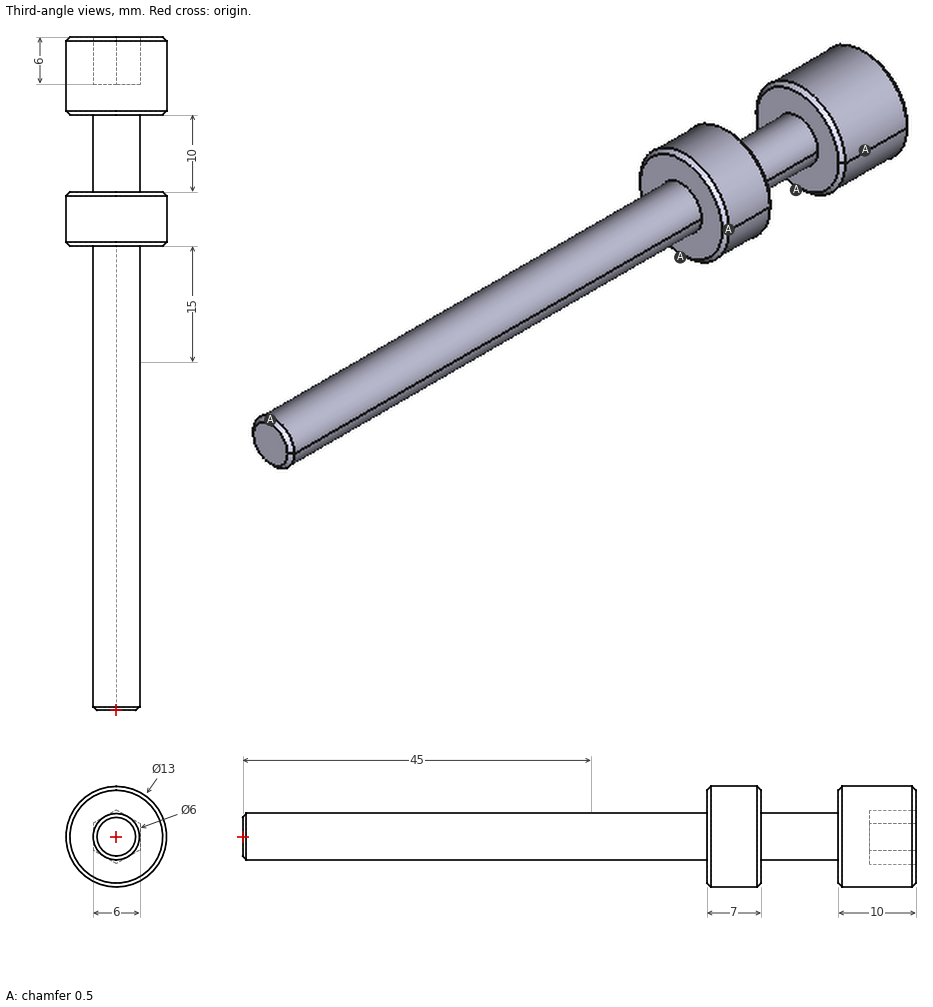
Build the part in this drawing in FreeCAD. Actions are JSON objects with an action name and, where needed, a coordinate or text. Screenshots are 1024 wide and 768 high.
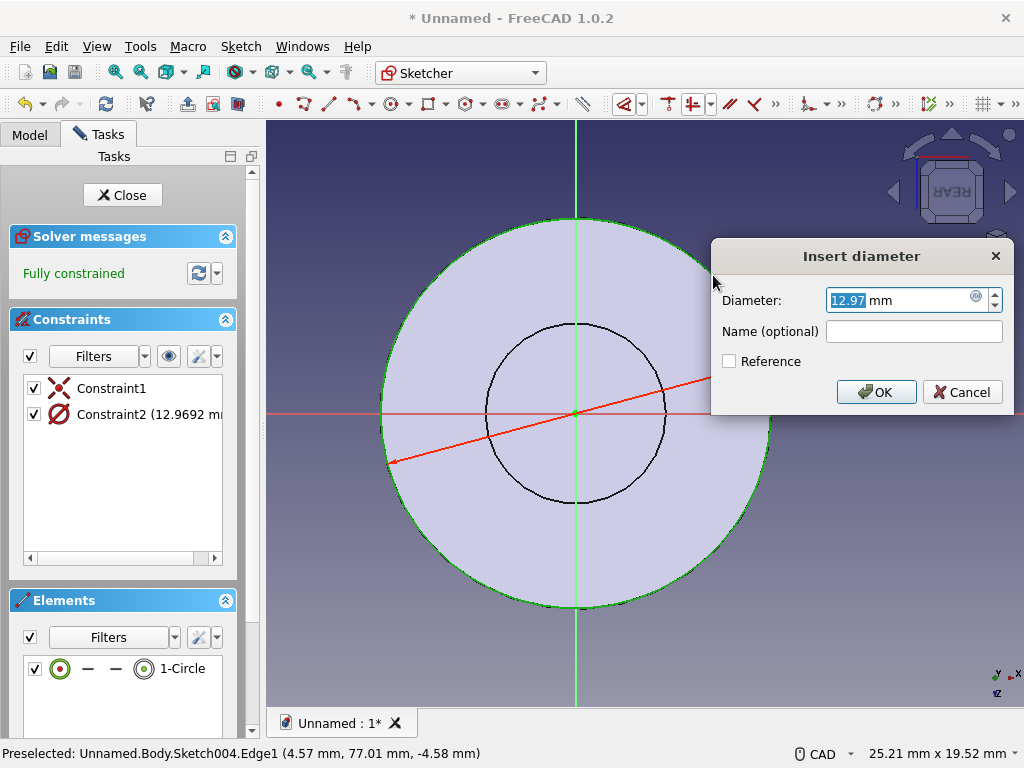
{"action": "type", "text": "13"}
{"action": "key", "text": "Return"}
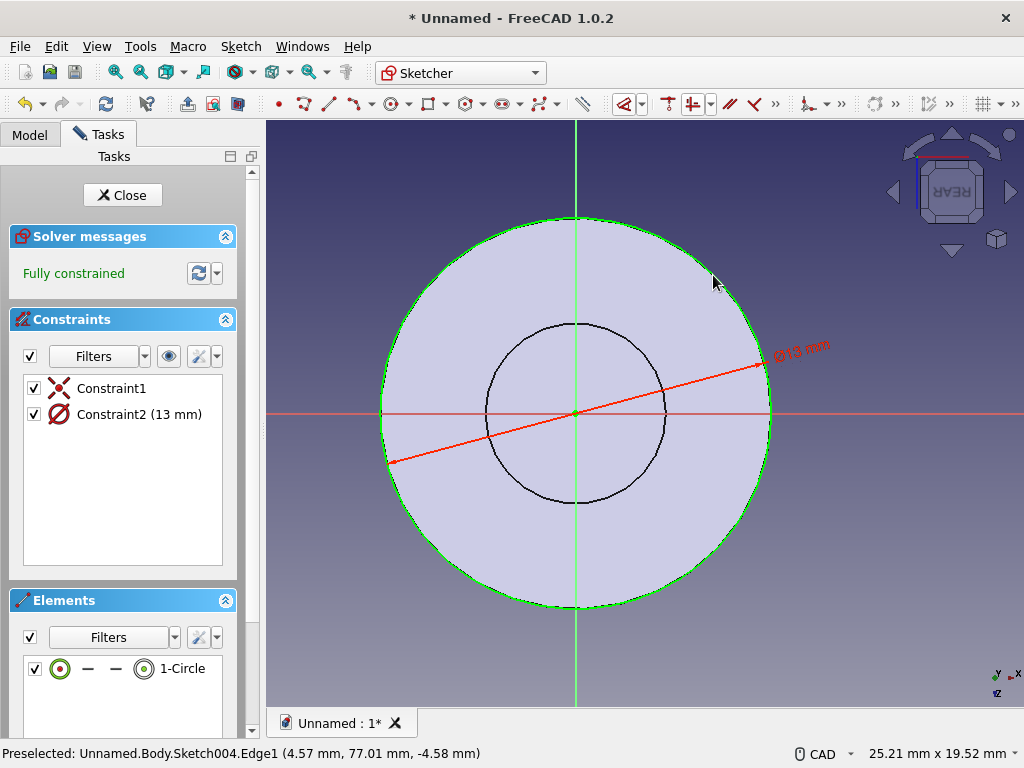
{"action": "left_click", "coordinate": [123, 195]}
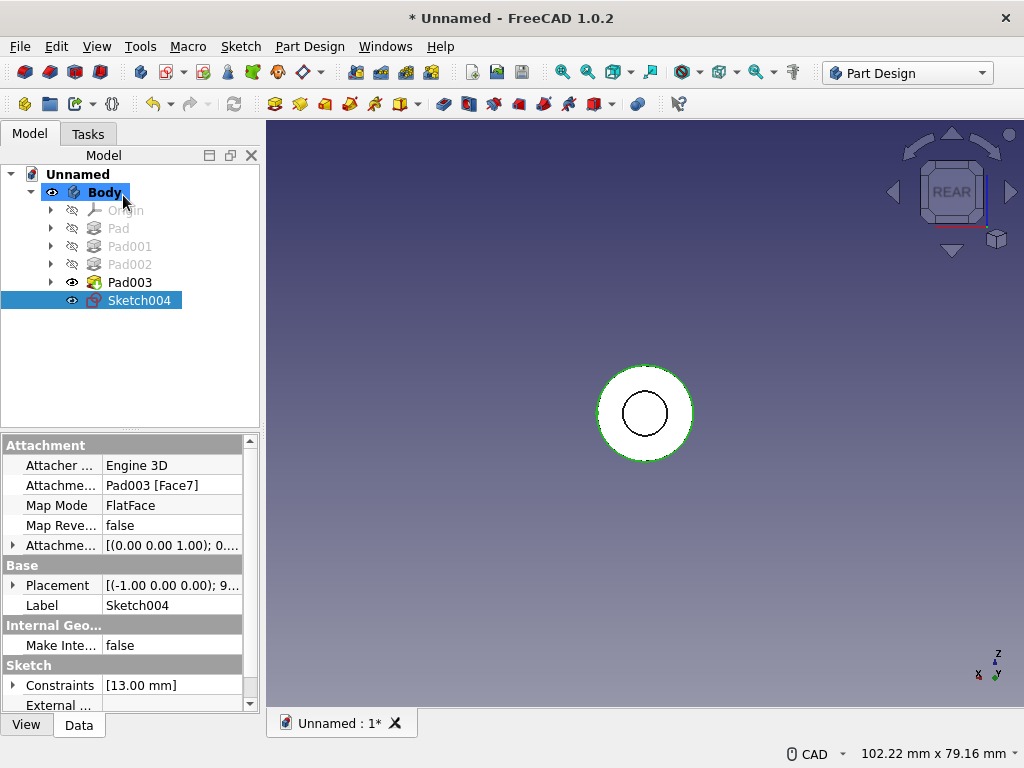
{"action": "left_click", "coordinate": [275, 104]}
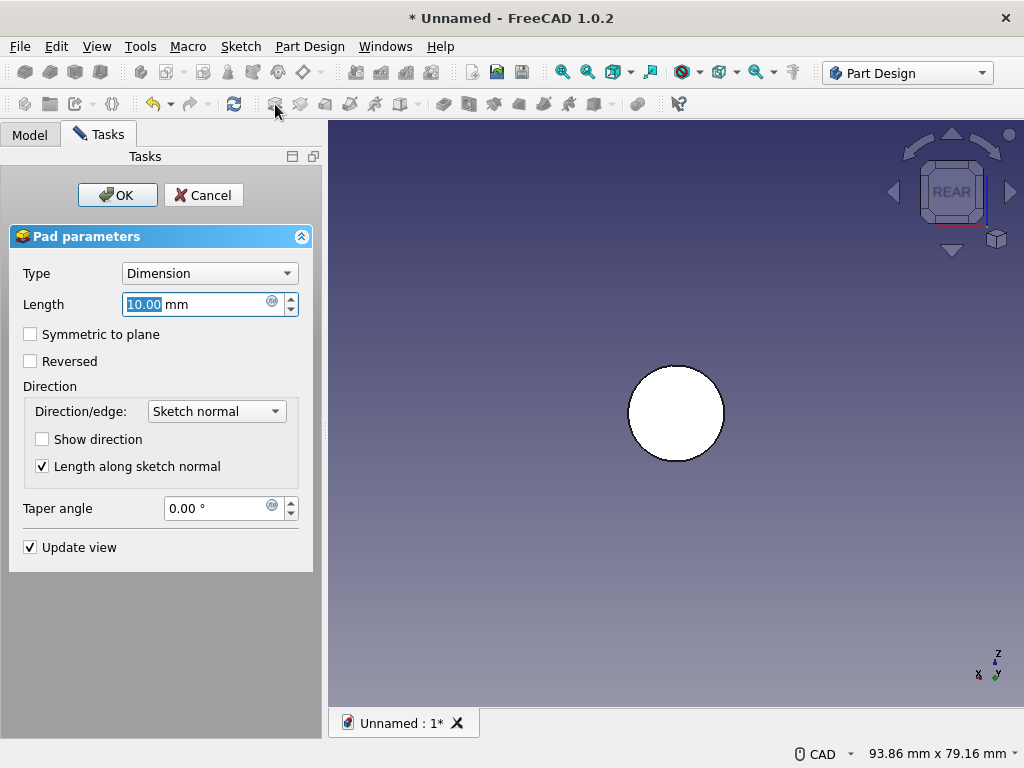
{"action": "type", "text": "10"}
{"action": "key", "text": "Tab"}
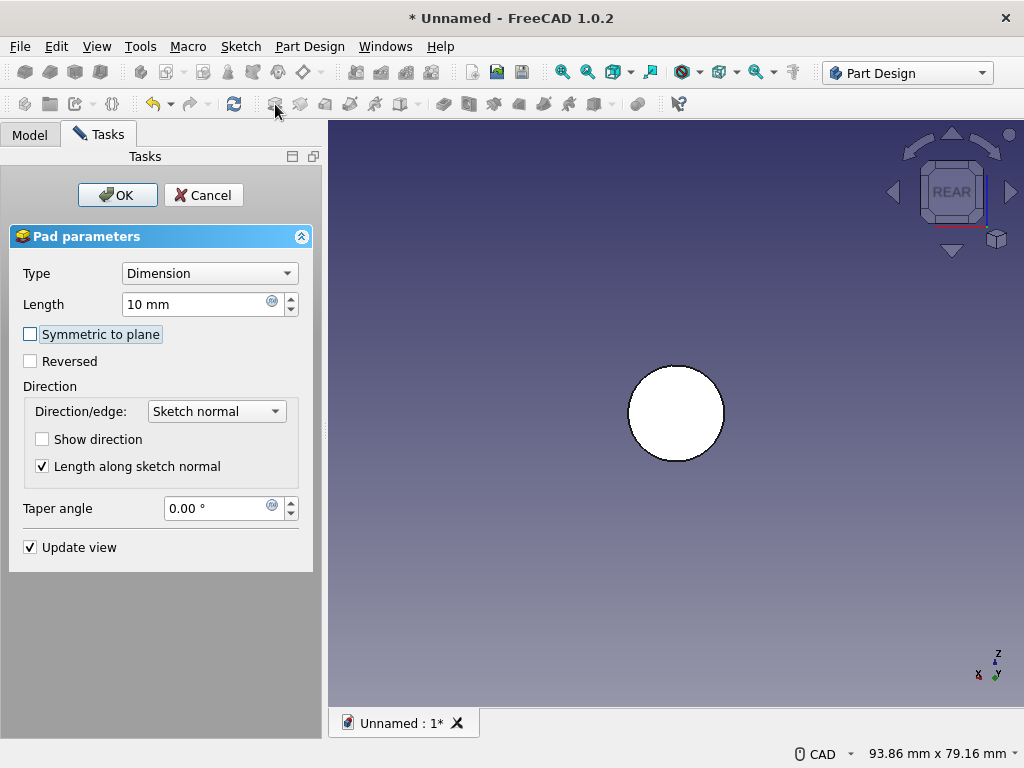
{"action": "left_click", "coordinate": [118, 195]}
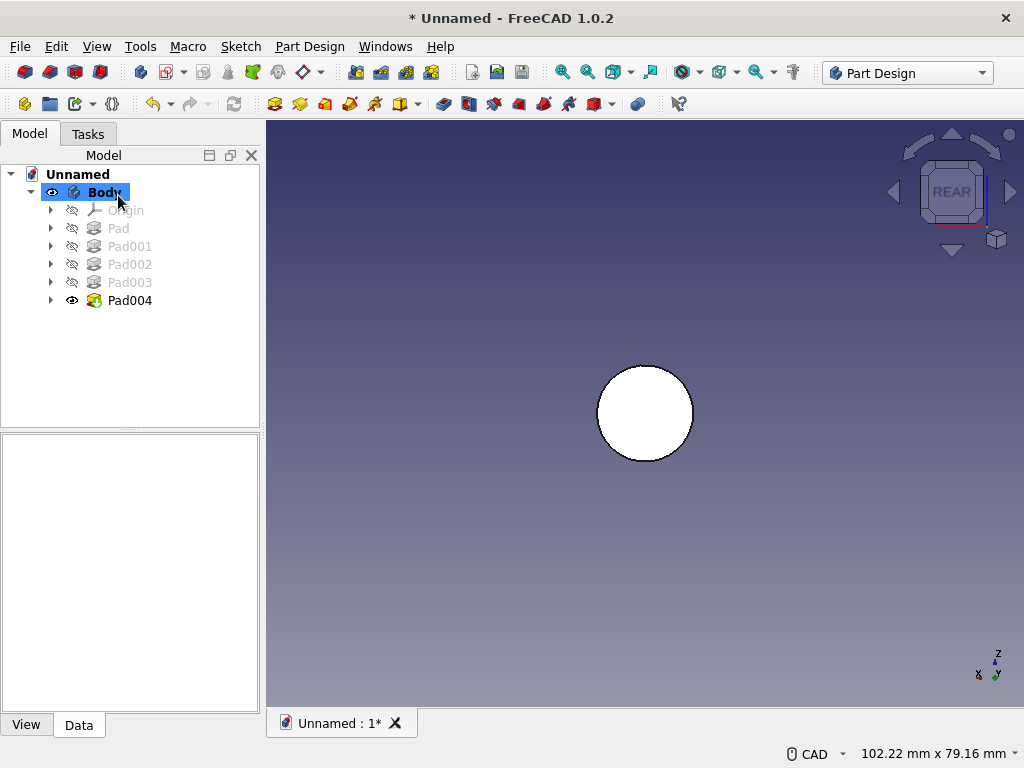
{"action": "left_click", "coordinate": [563, 72]}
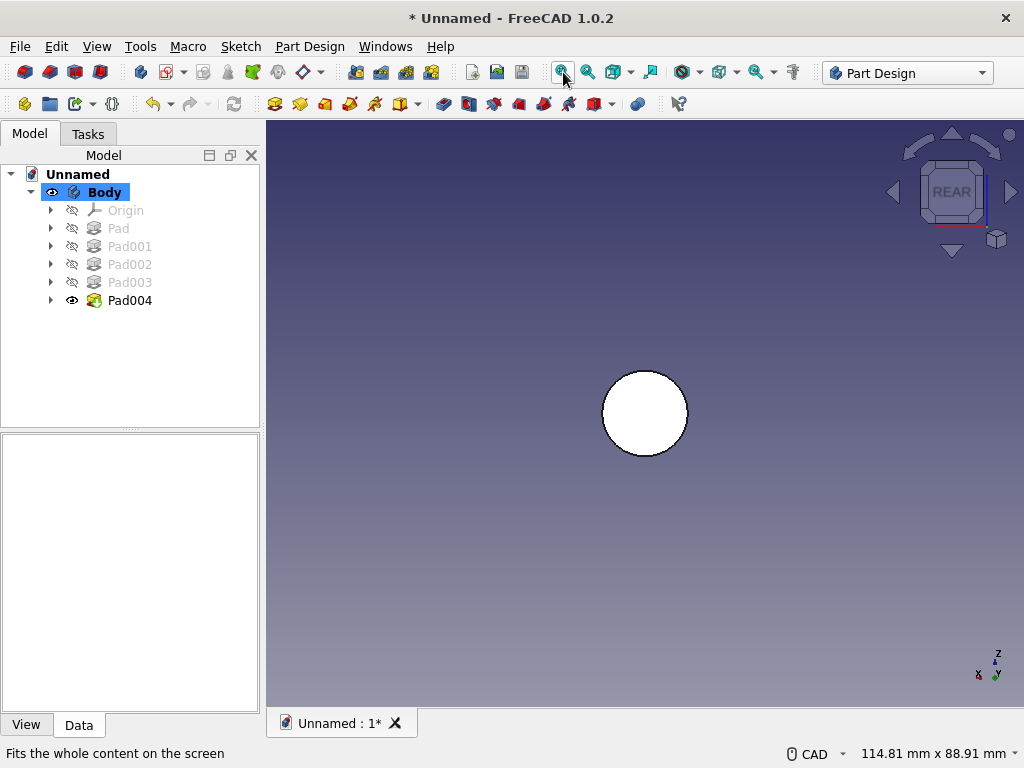
{"action": "left_click", "coordinate": [645, 412]}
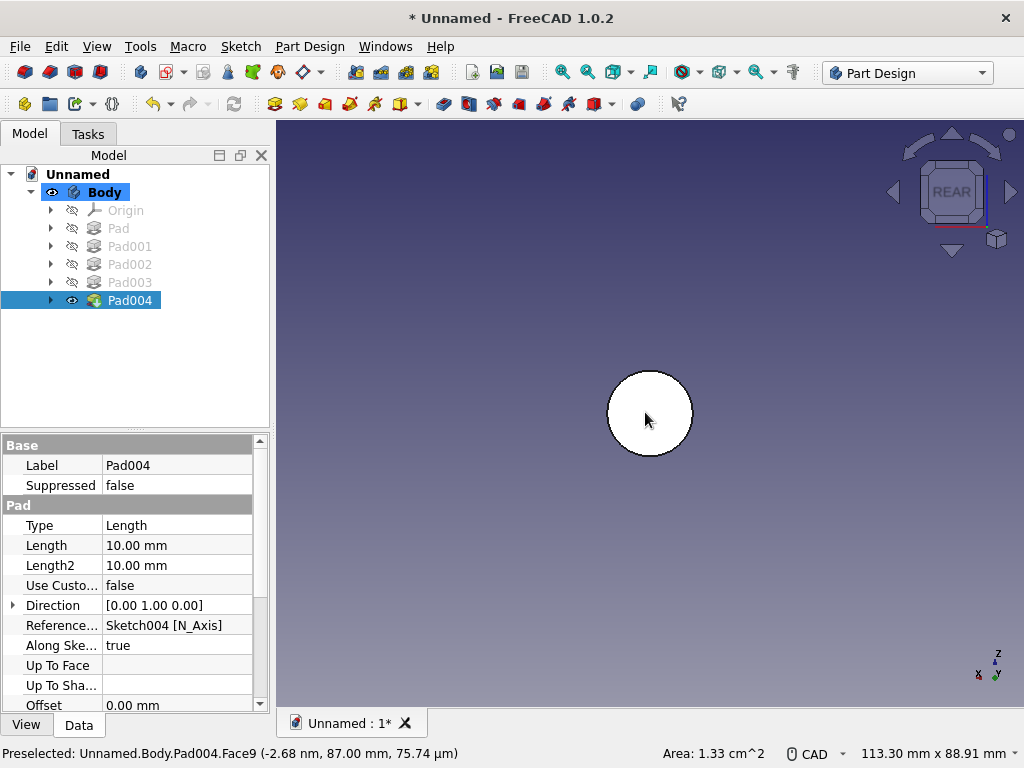
{"action": "left_click", "coordinate": [166, 72]}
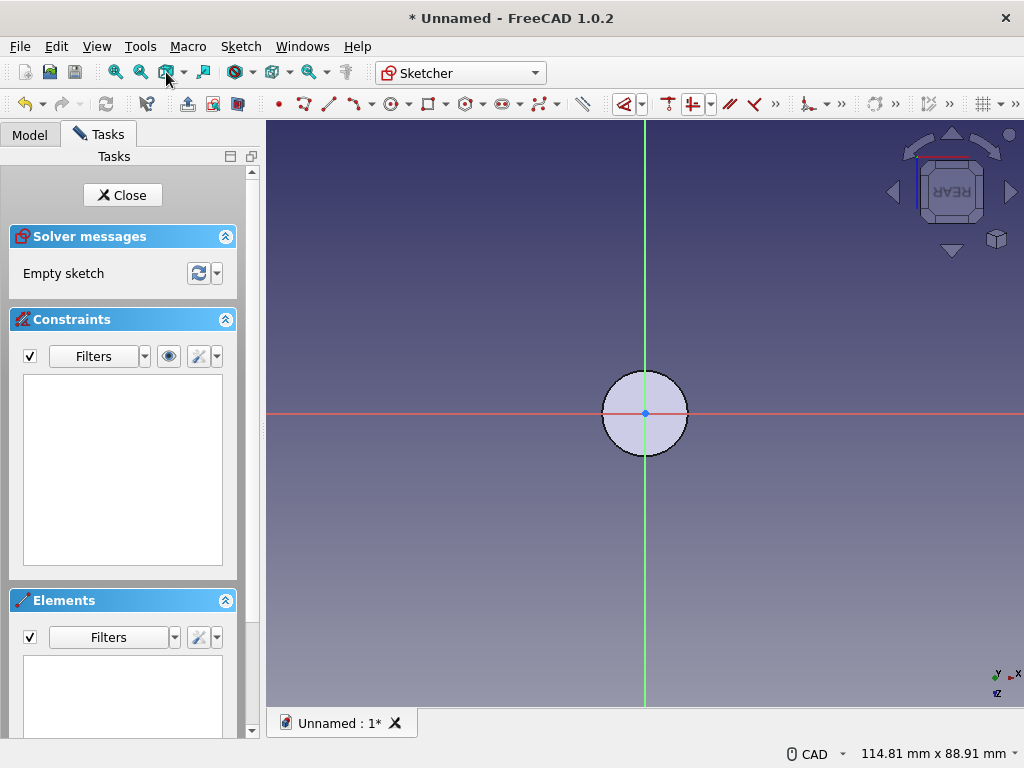
{"action": "scroll", "coordinate": [654, 413], "scroll_direction": "up", "scroll_amount": 11}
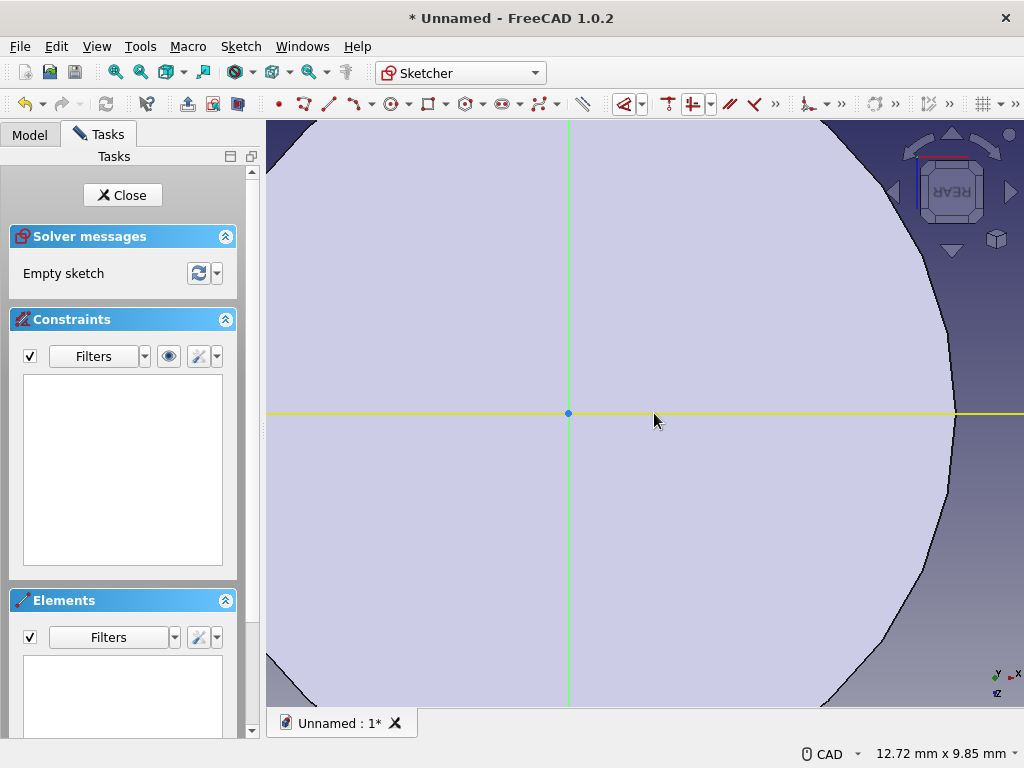
{"action": "left_click", "coordinate": [464, 104]}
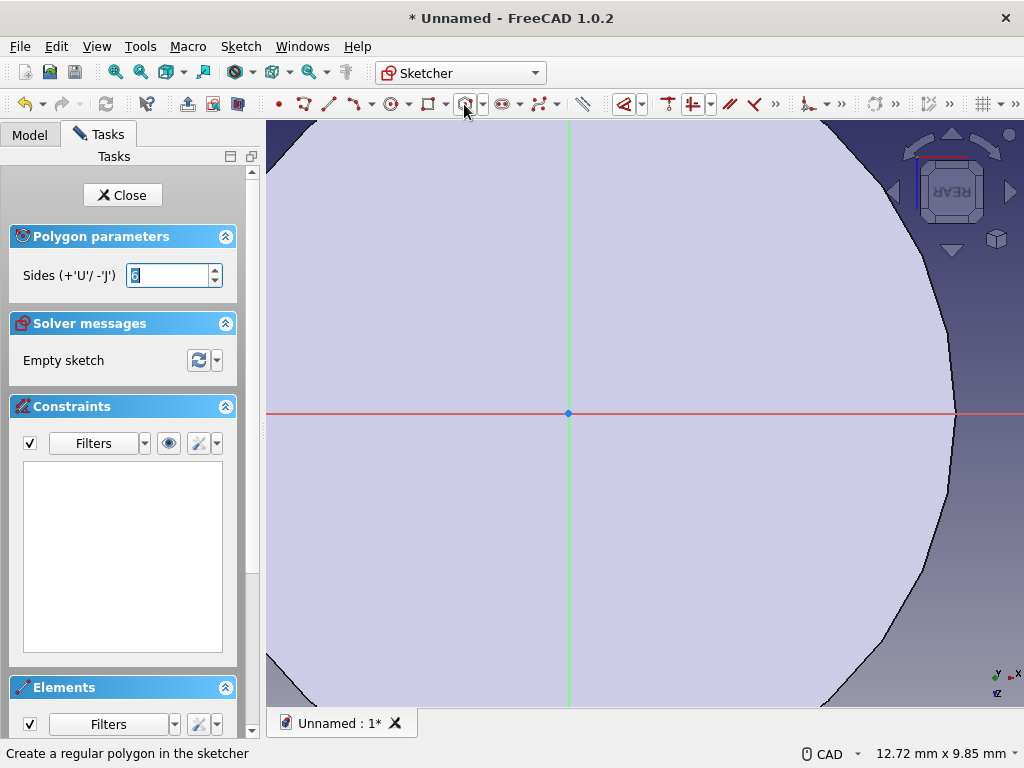
{"action": "left_click", "coordinate": [569, 413]}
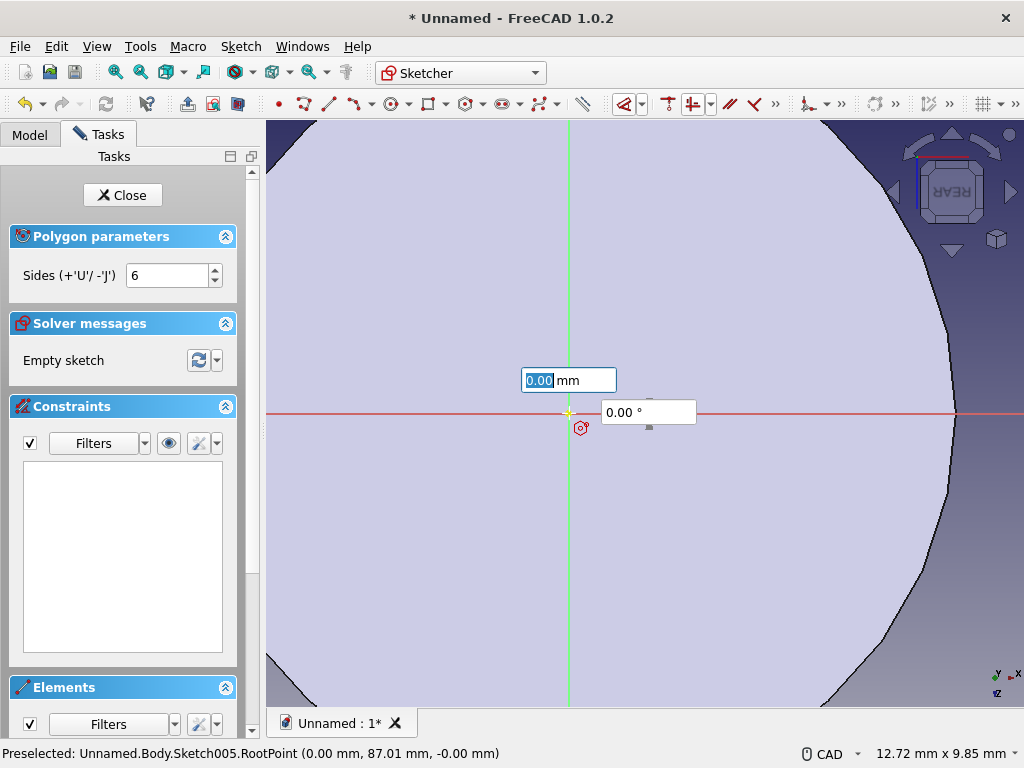
{"action": "left_click", "coordinate": [569, 207]}
{"action": "right_click", "coordinate": [569, 207]}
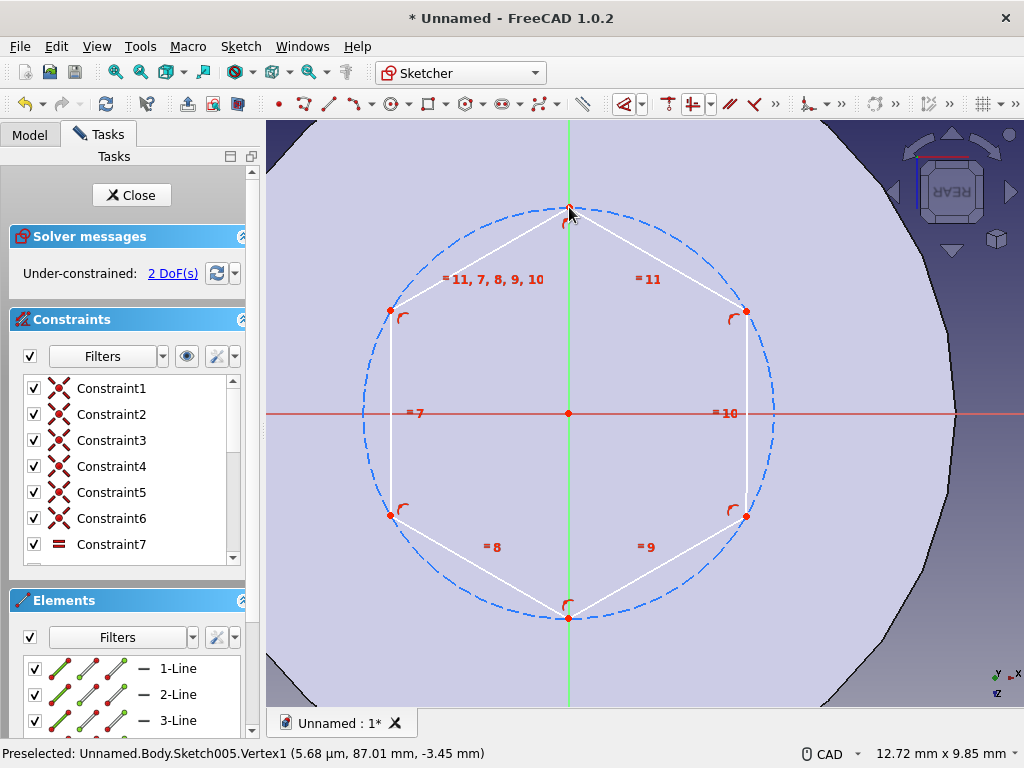
{"action": "left_click", "coordinate": [391, 372]}